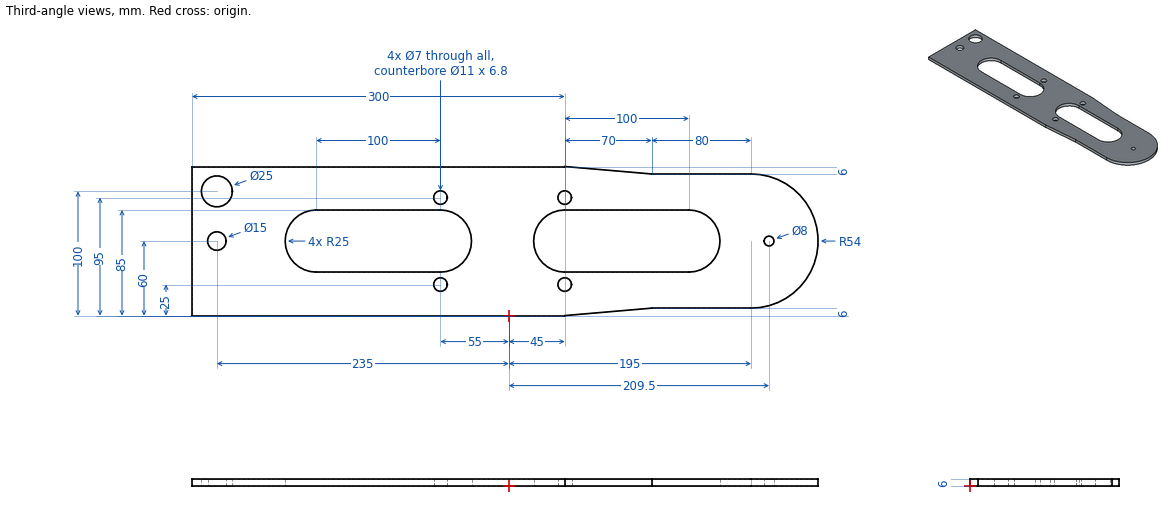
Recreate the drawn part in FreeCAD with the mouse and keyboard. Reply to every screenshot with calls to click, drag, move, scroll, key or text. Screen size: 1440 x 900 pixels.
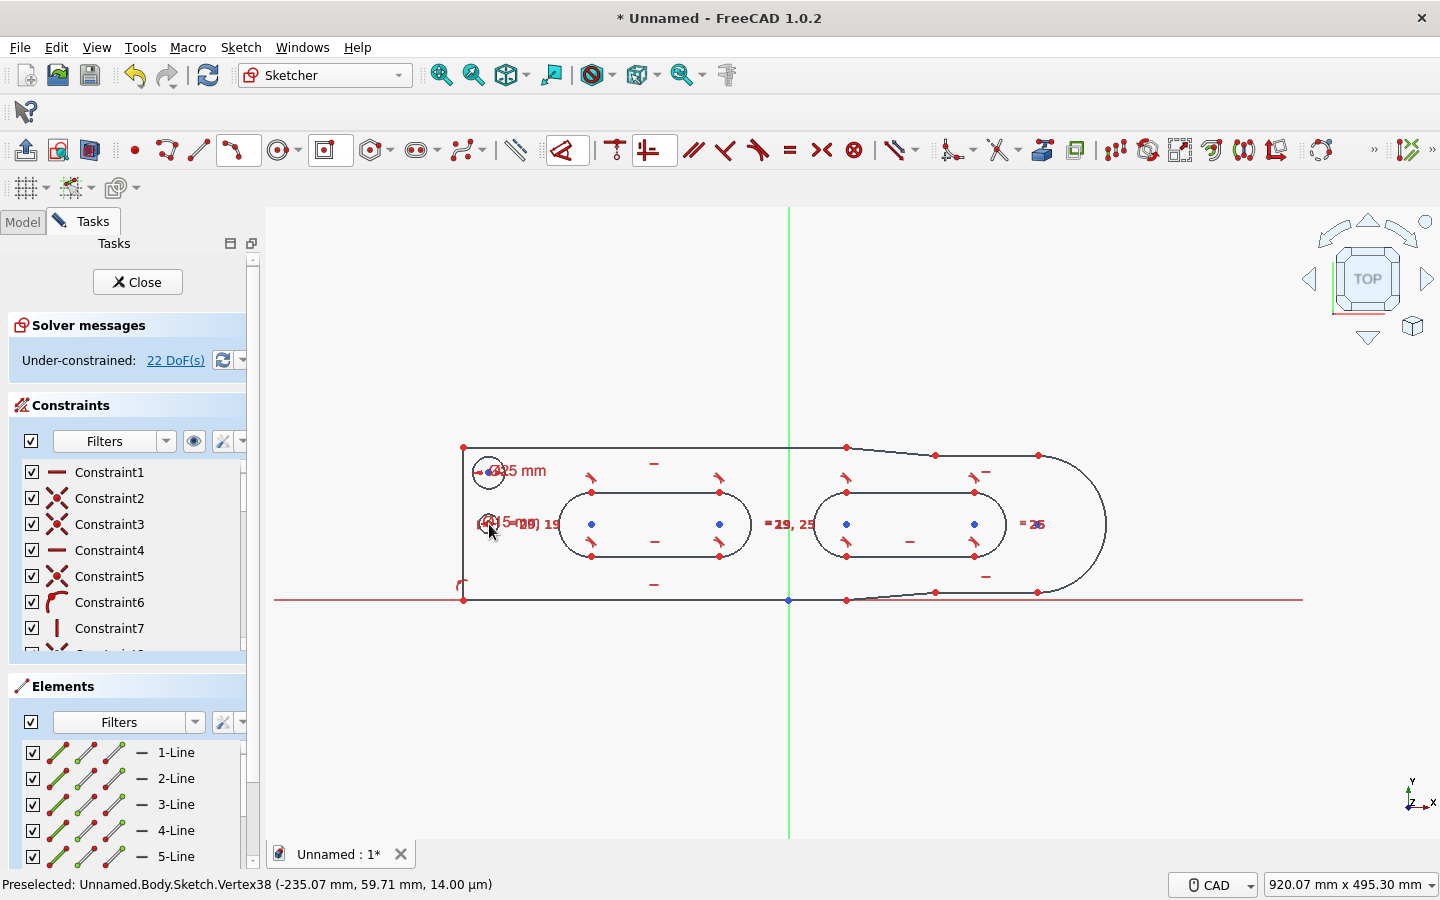
click(489, 473)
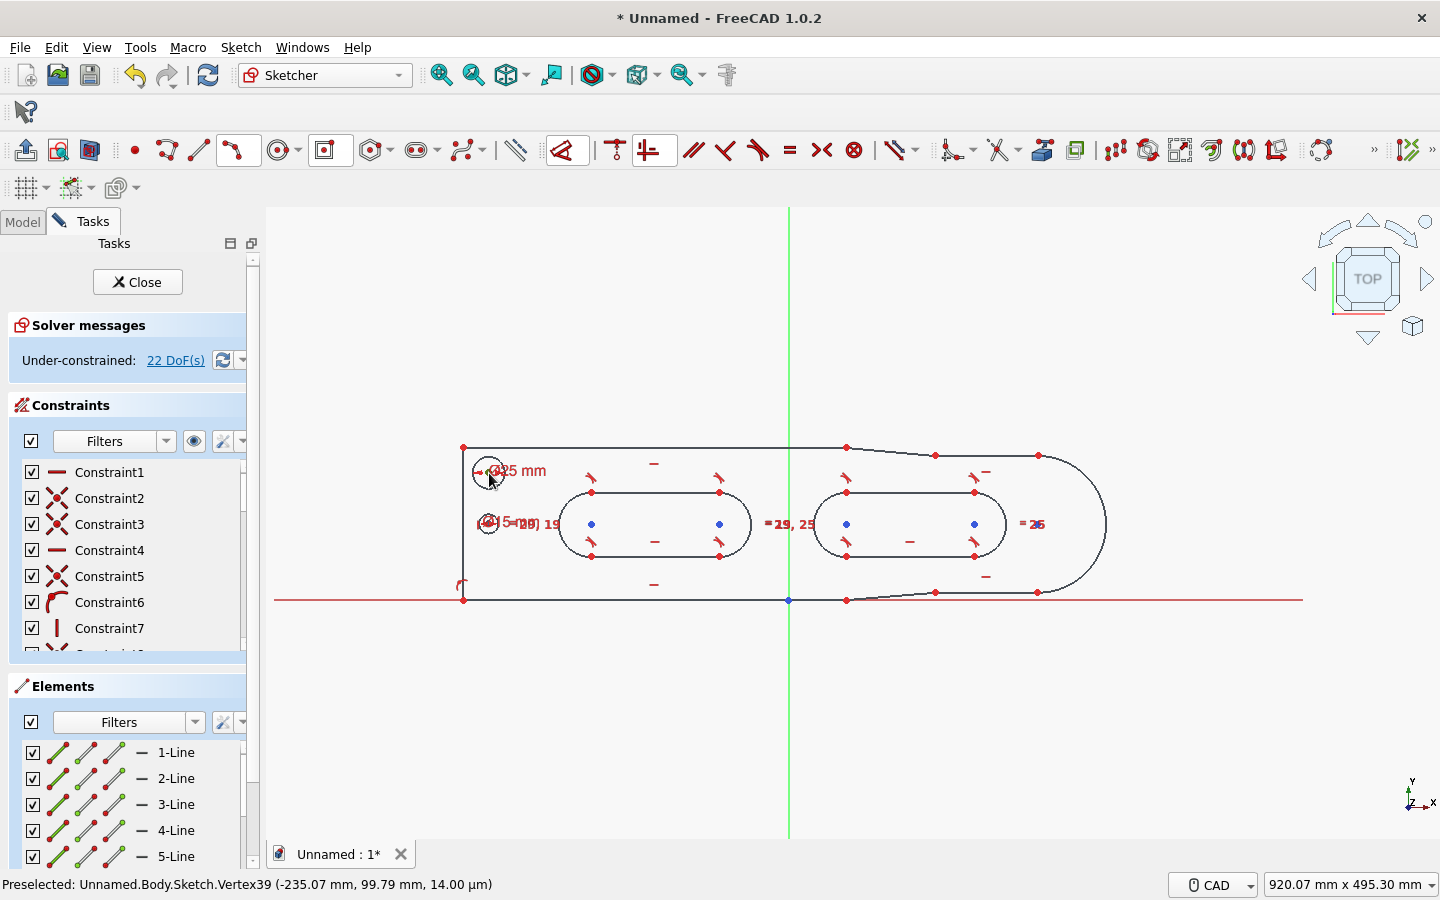
key(v)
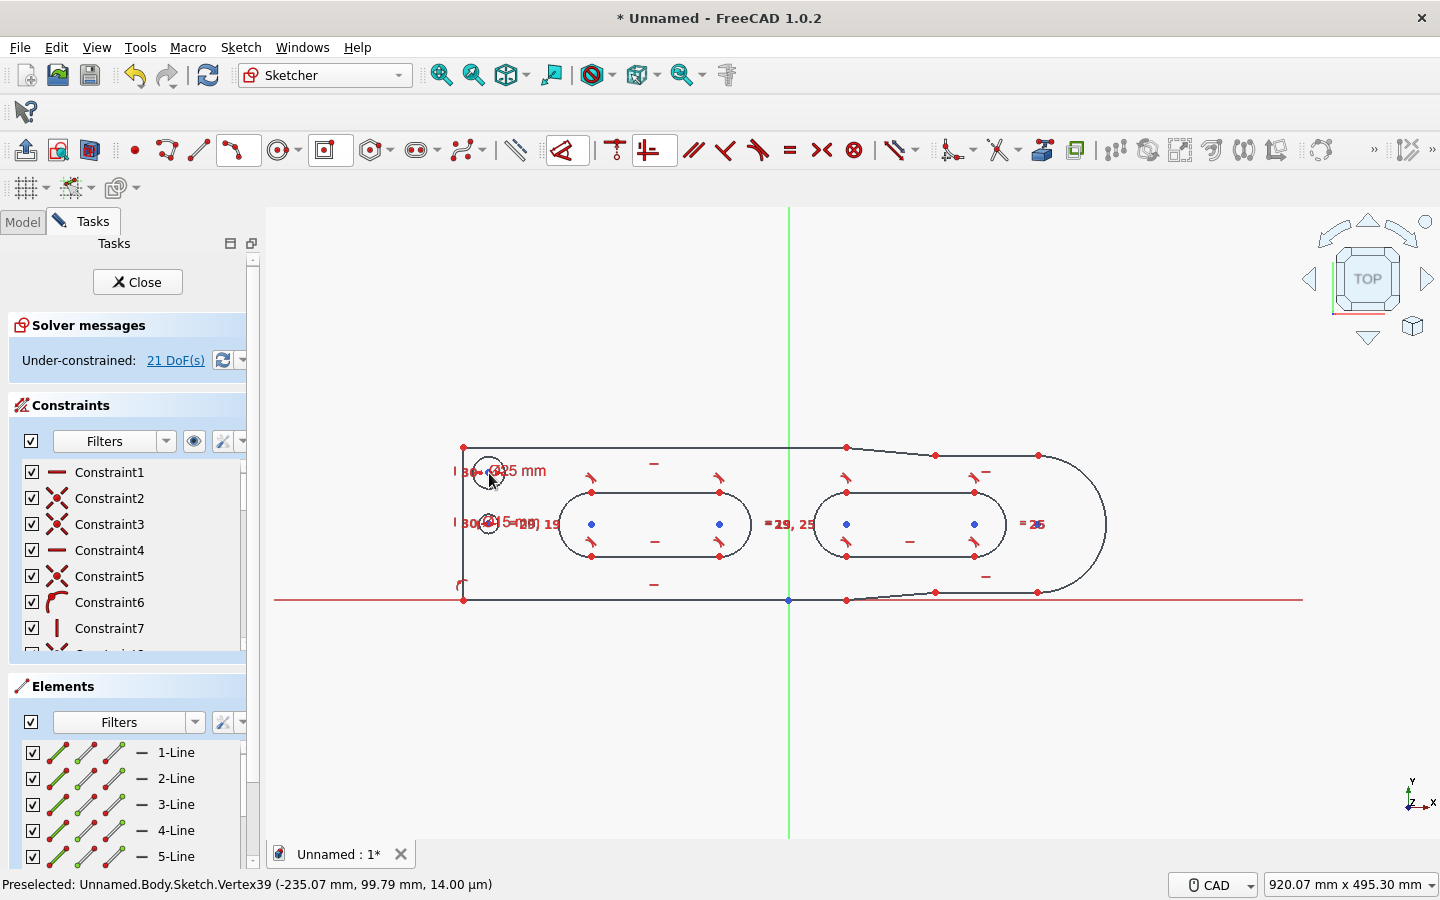
click(1093, 565)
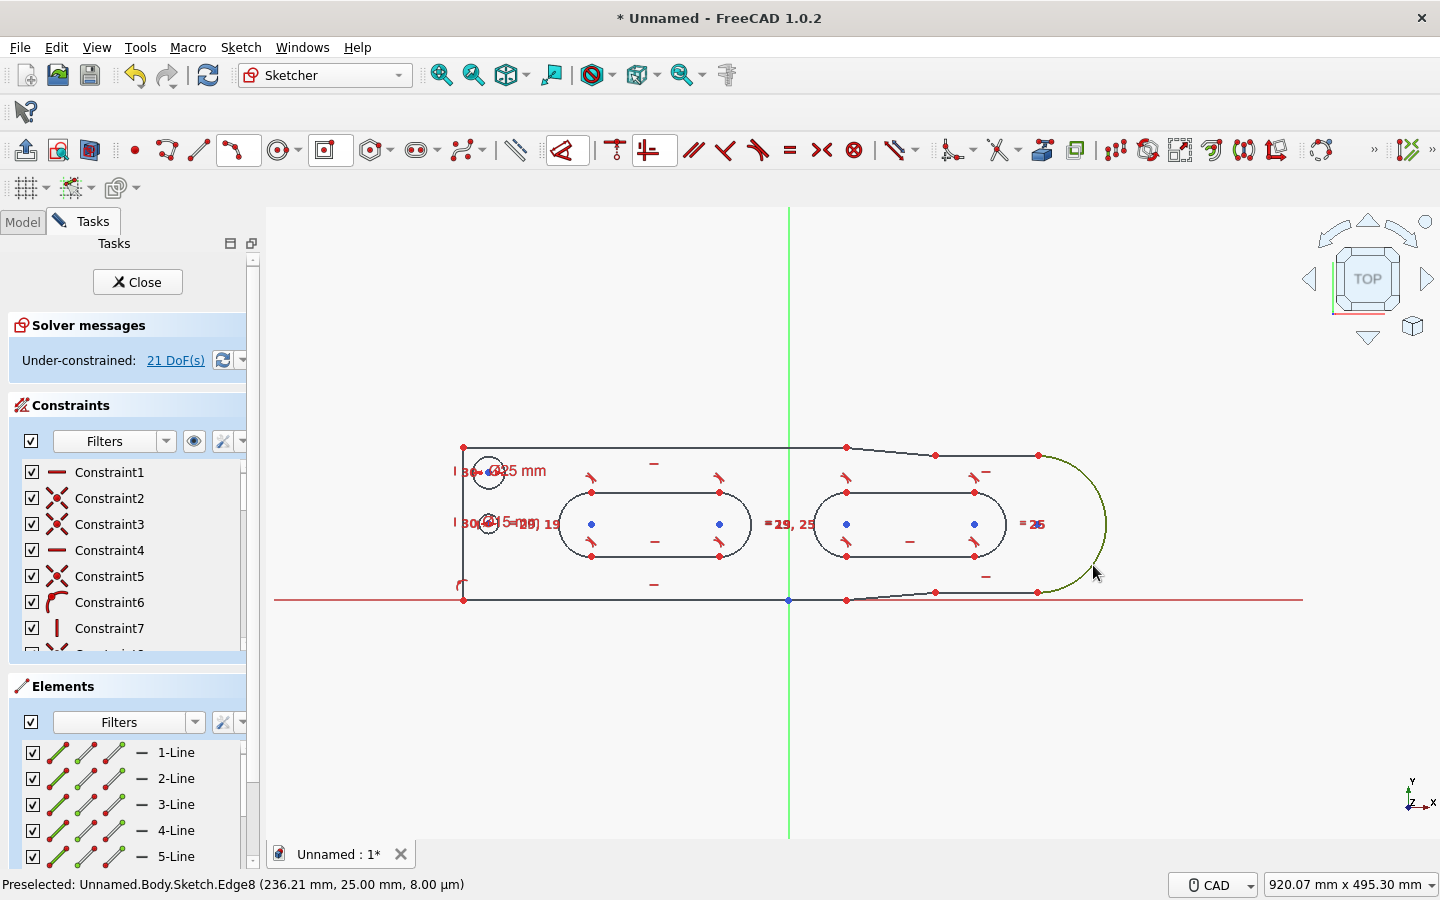
key(k)
key(r)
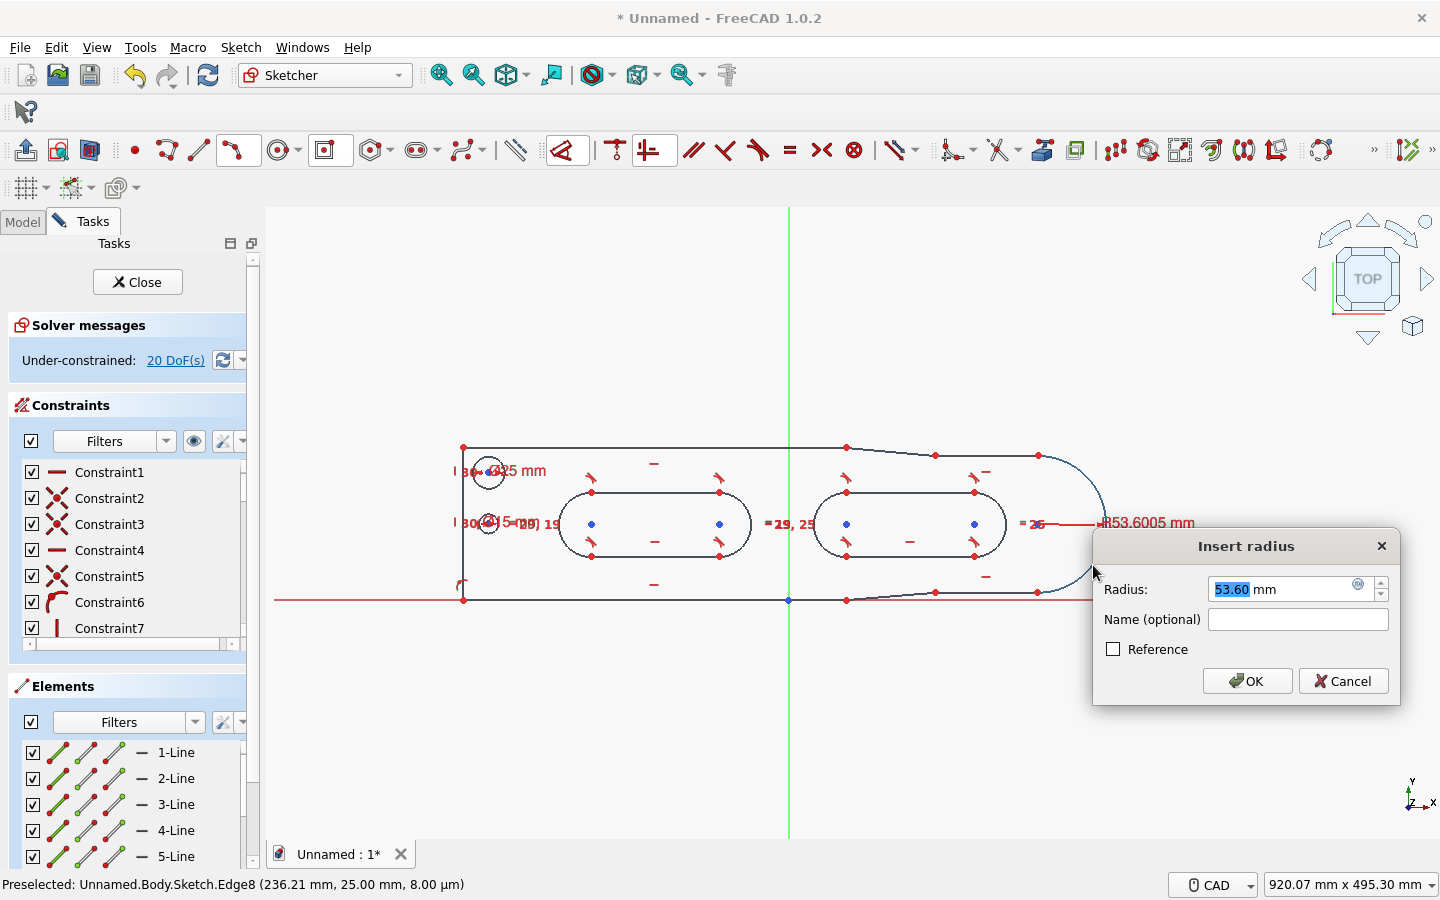
text(54)
key(Return)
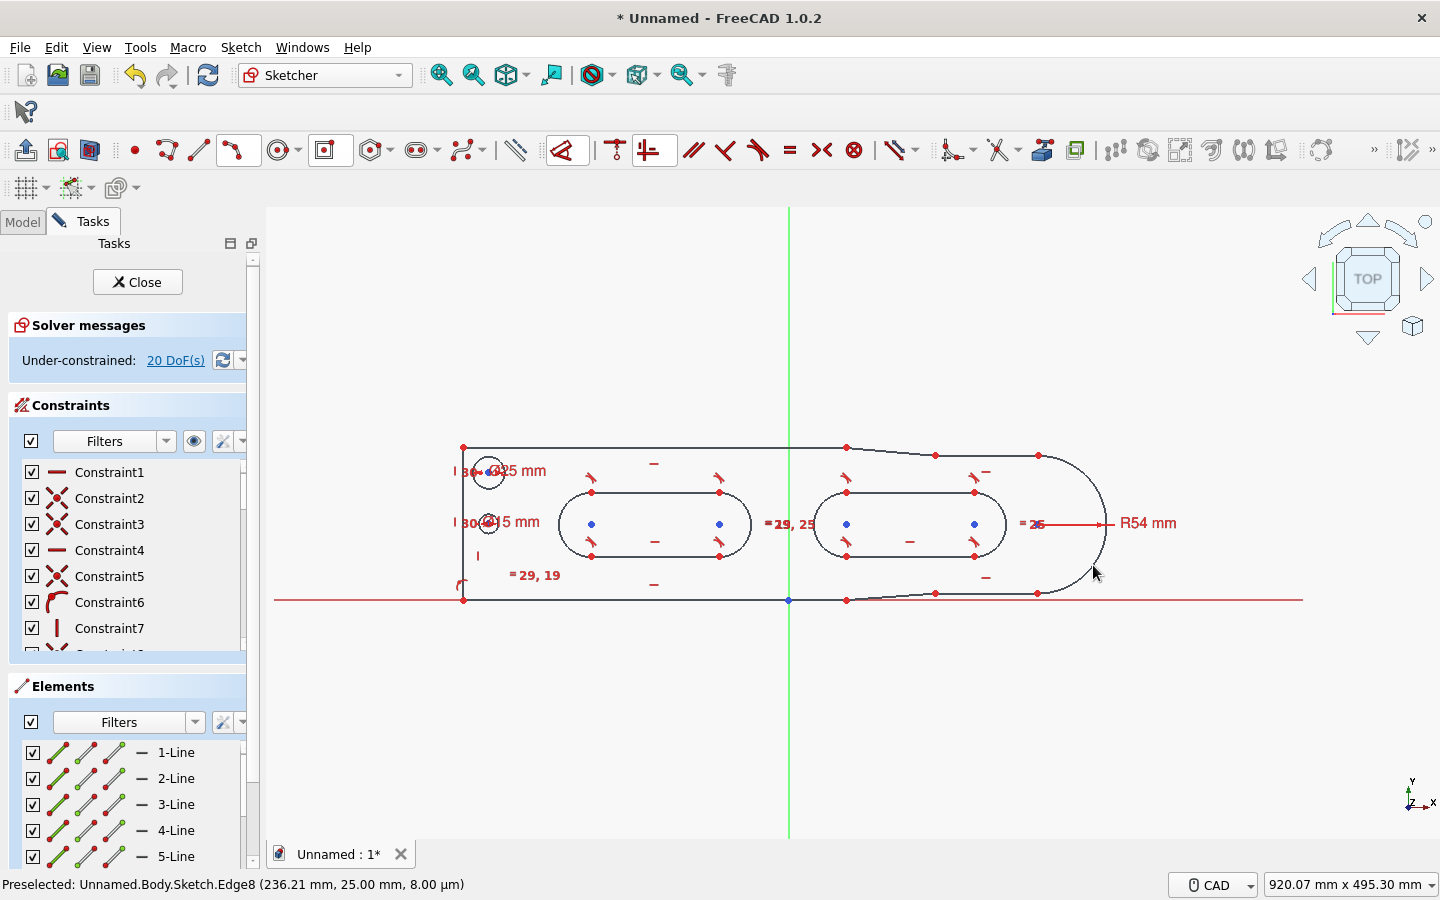
scroll(565, 506, up, 2)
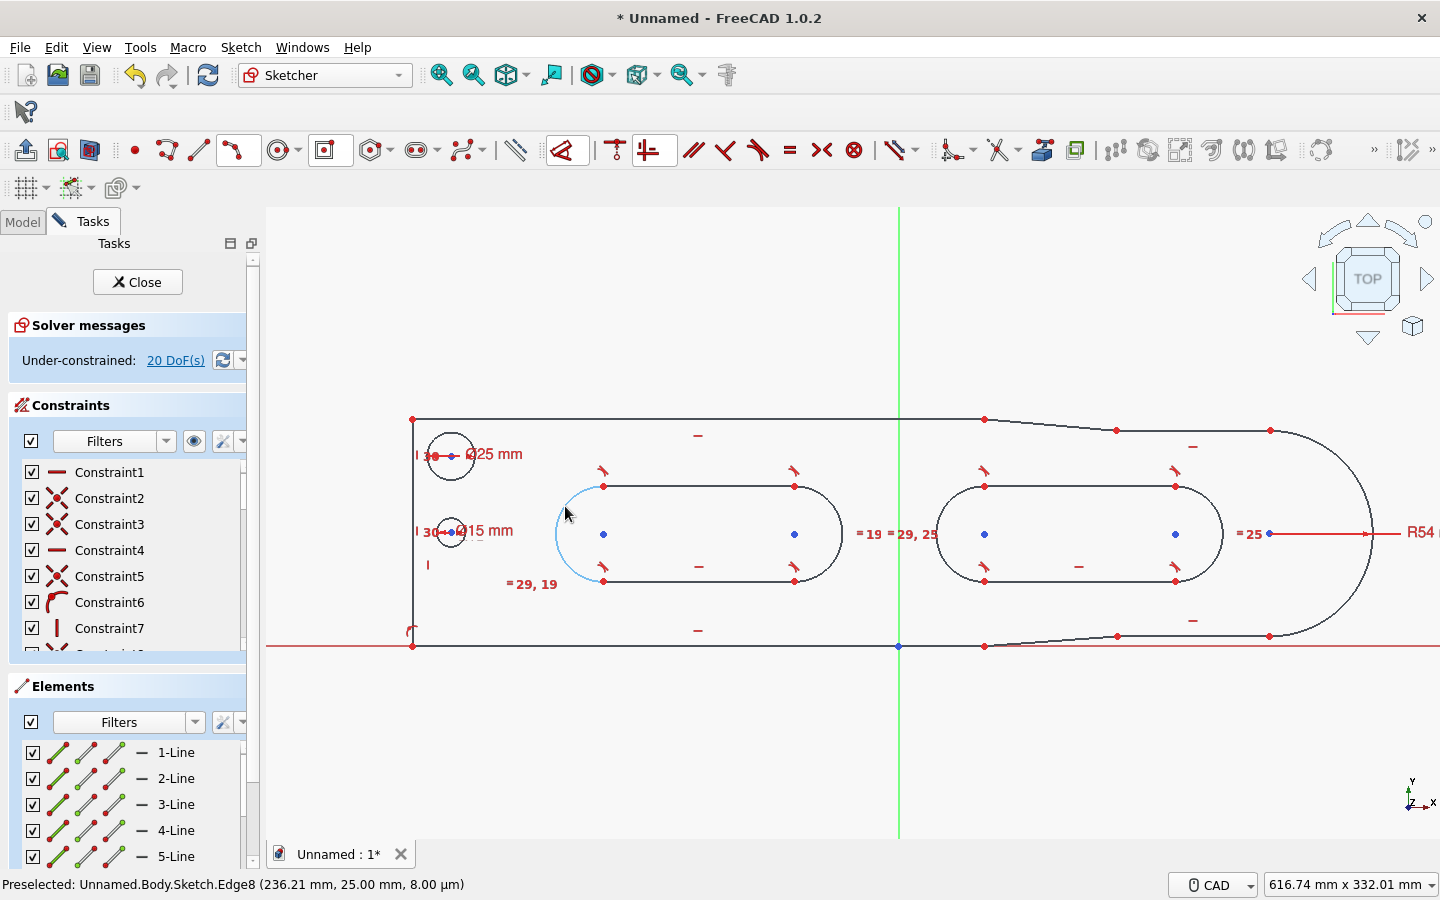
click(565, 506)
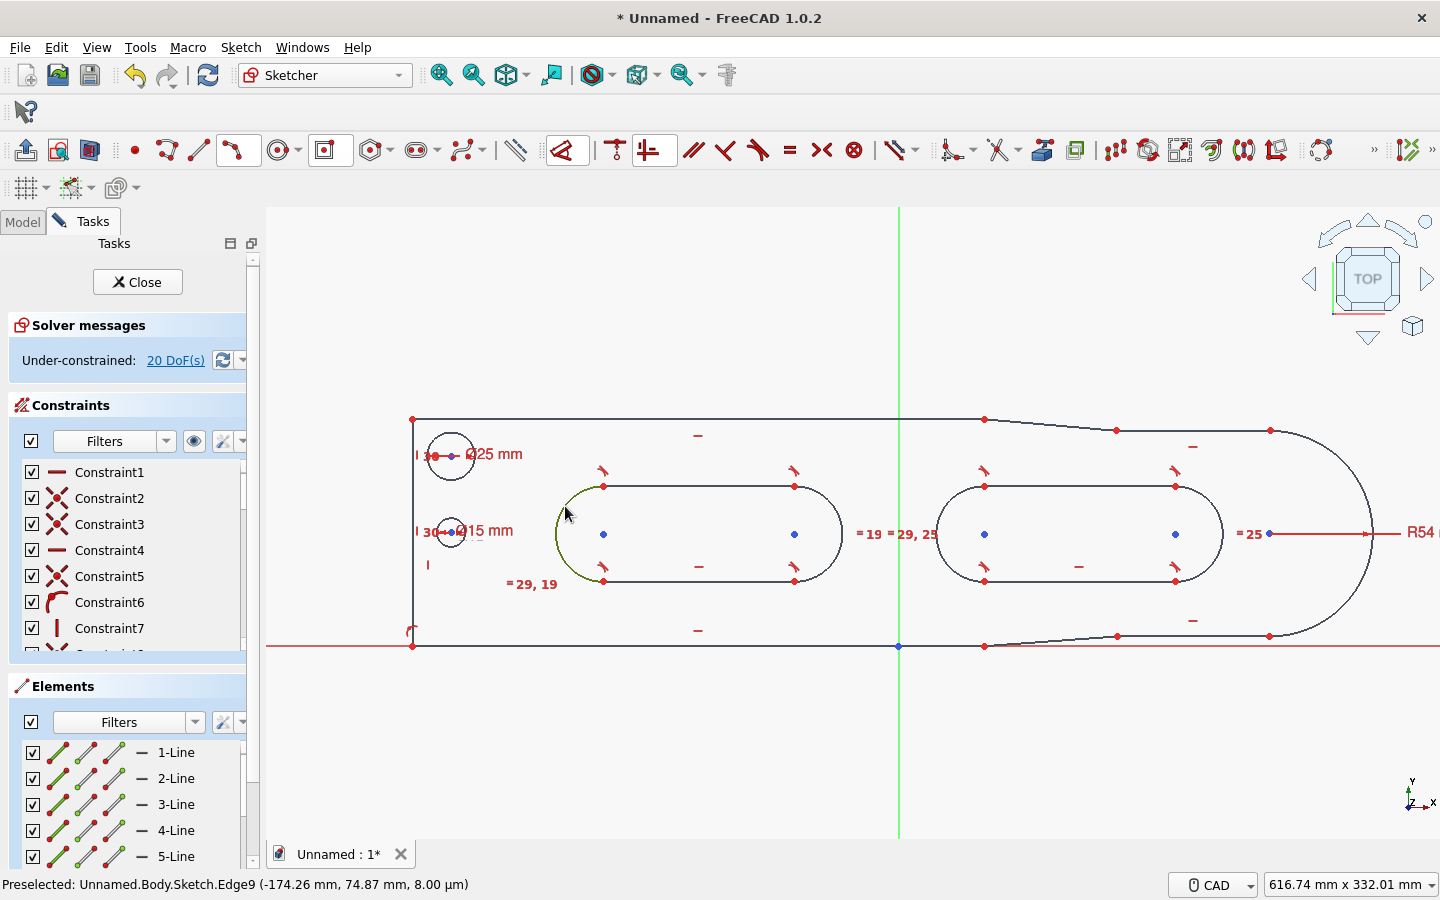
key(k)
key(r)